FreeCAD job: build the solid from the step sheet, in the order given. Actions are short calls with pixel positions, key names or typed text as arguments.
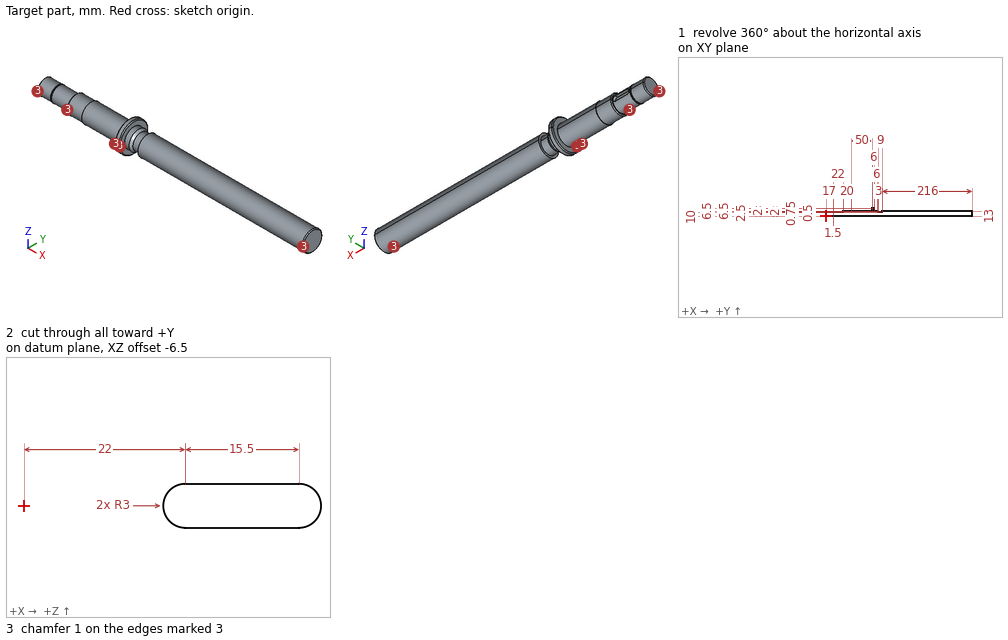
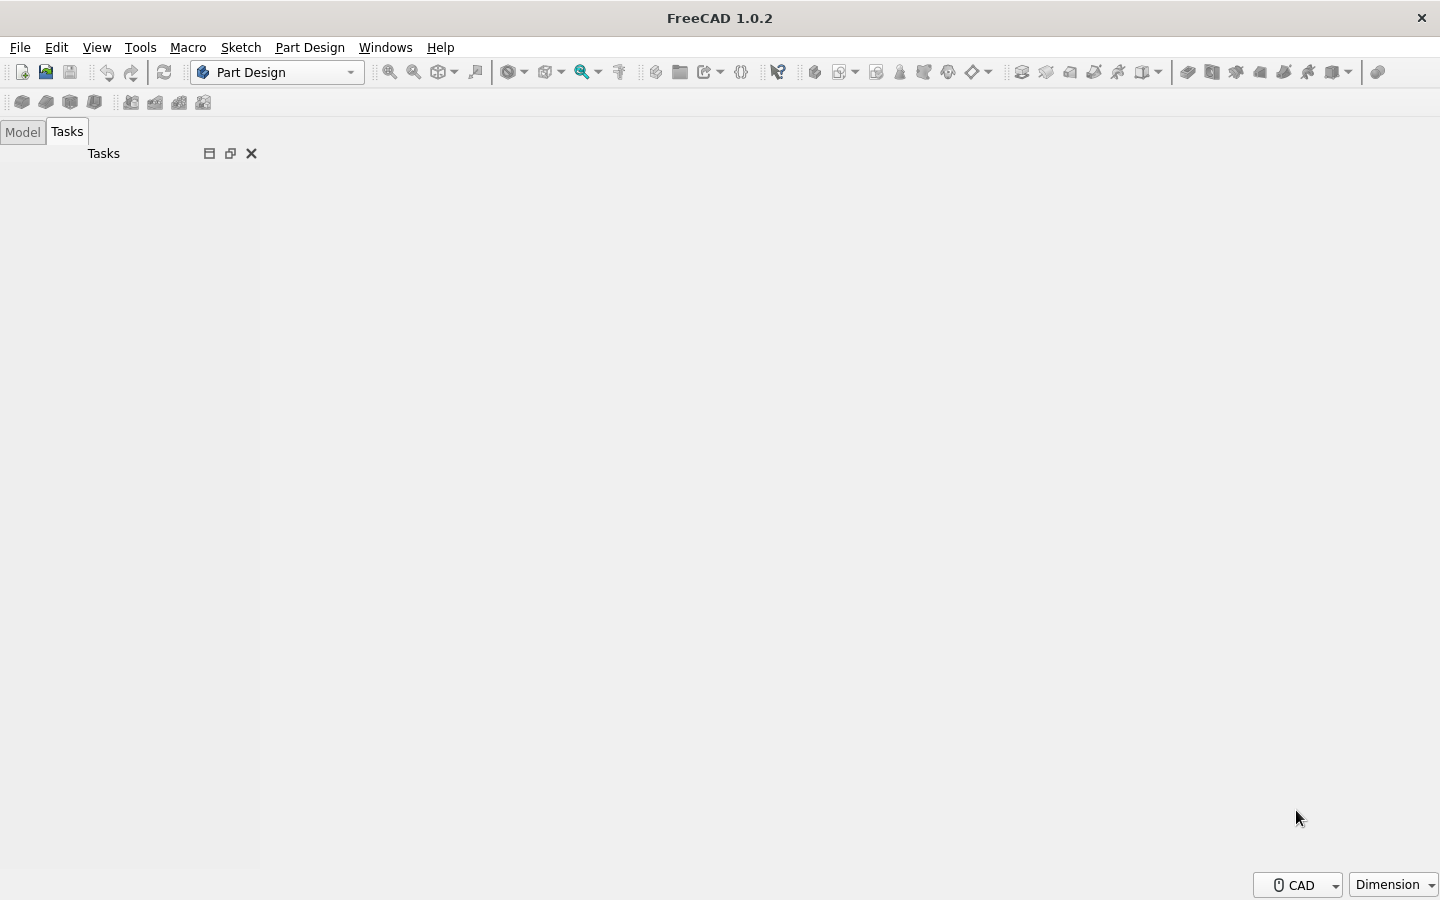
click(22, 72)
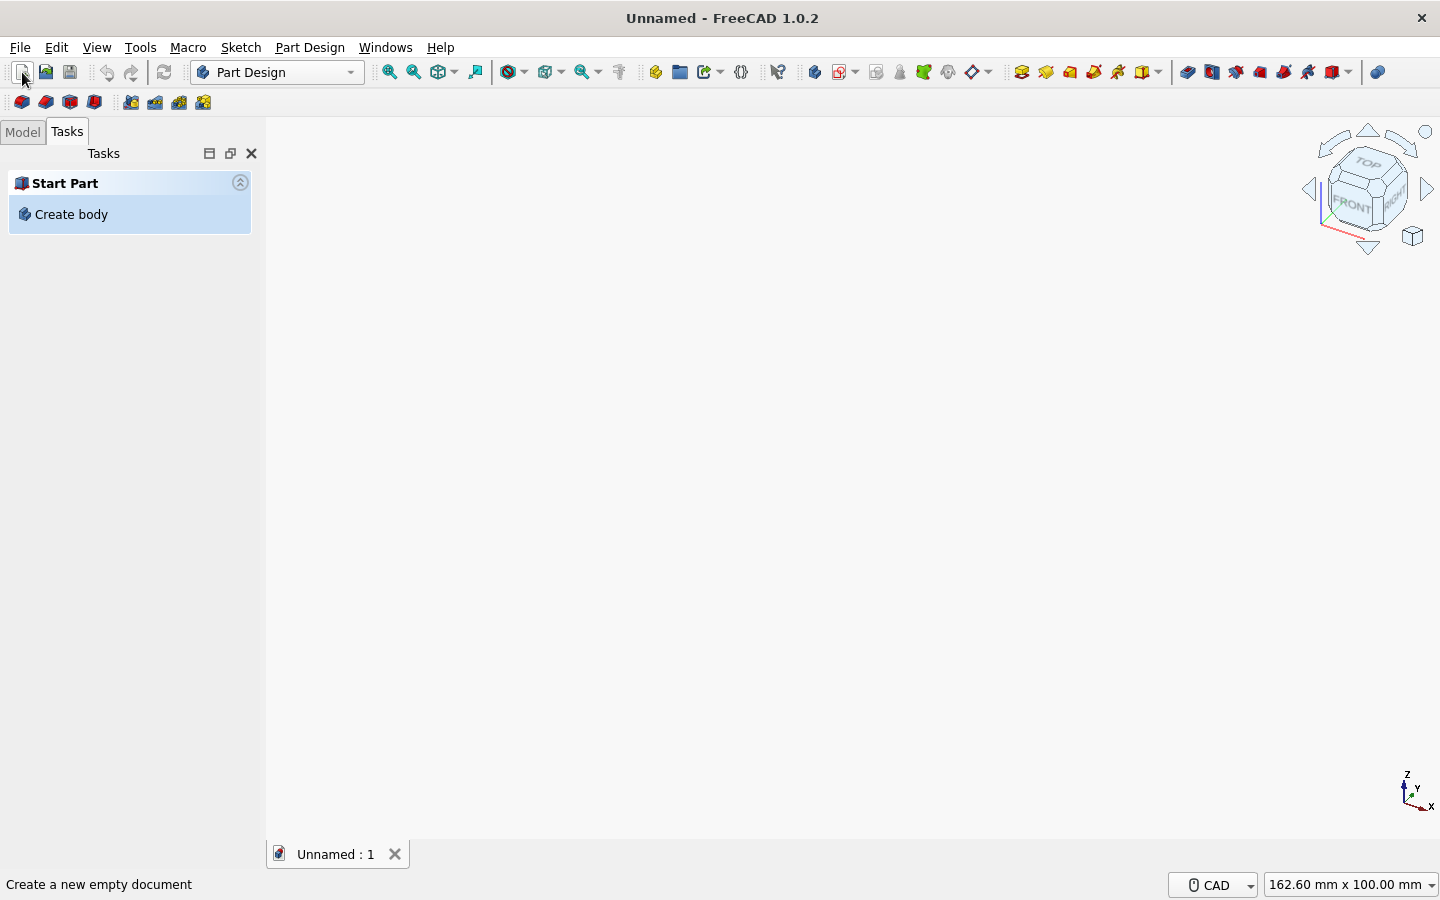
click(840, 72)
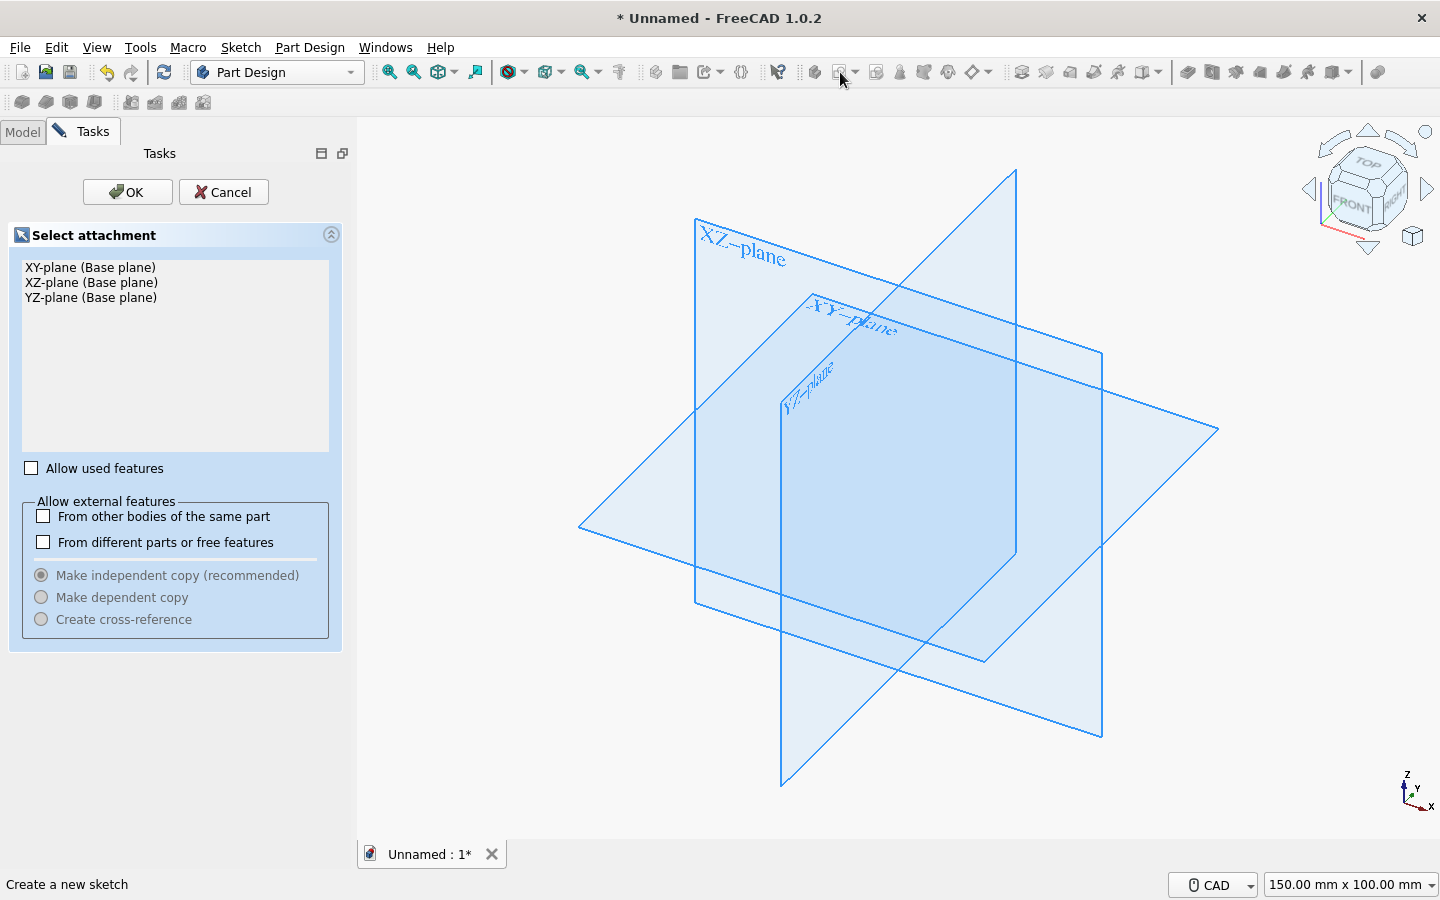
click(82, 268)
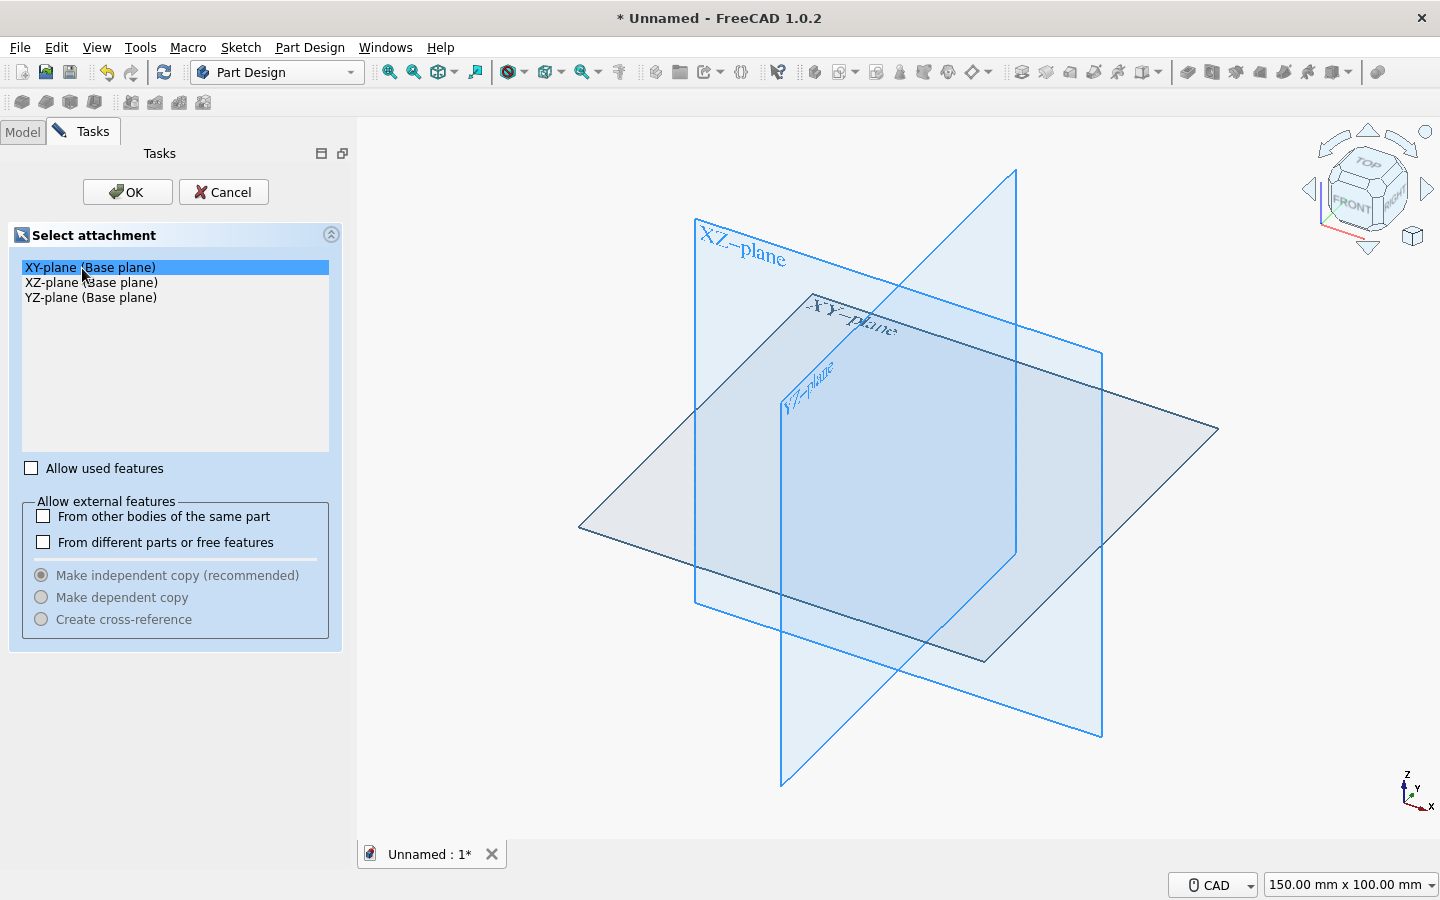
click(128, 192)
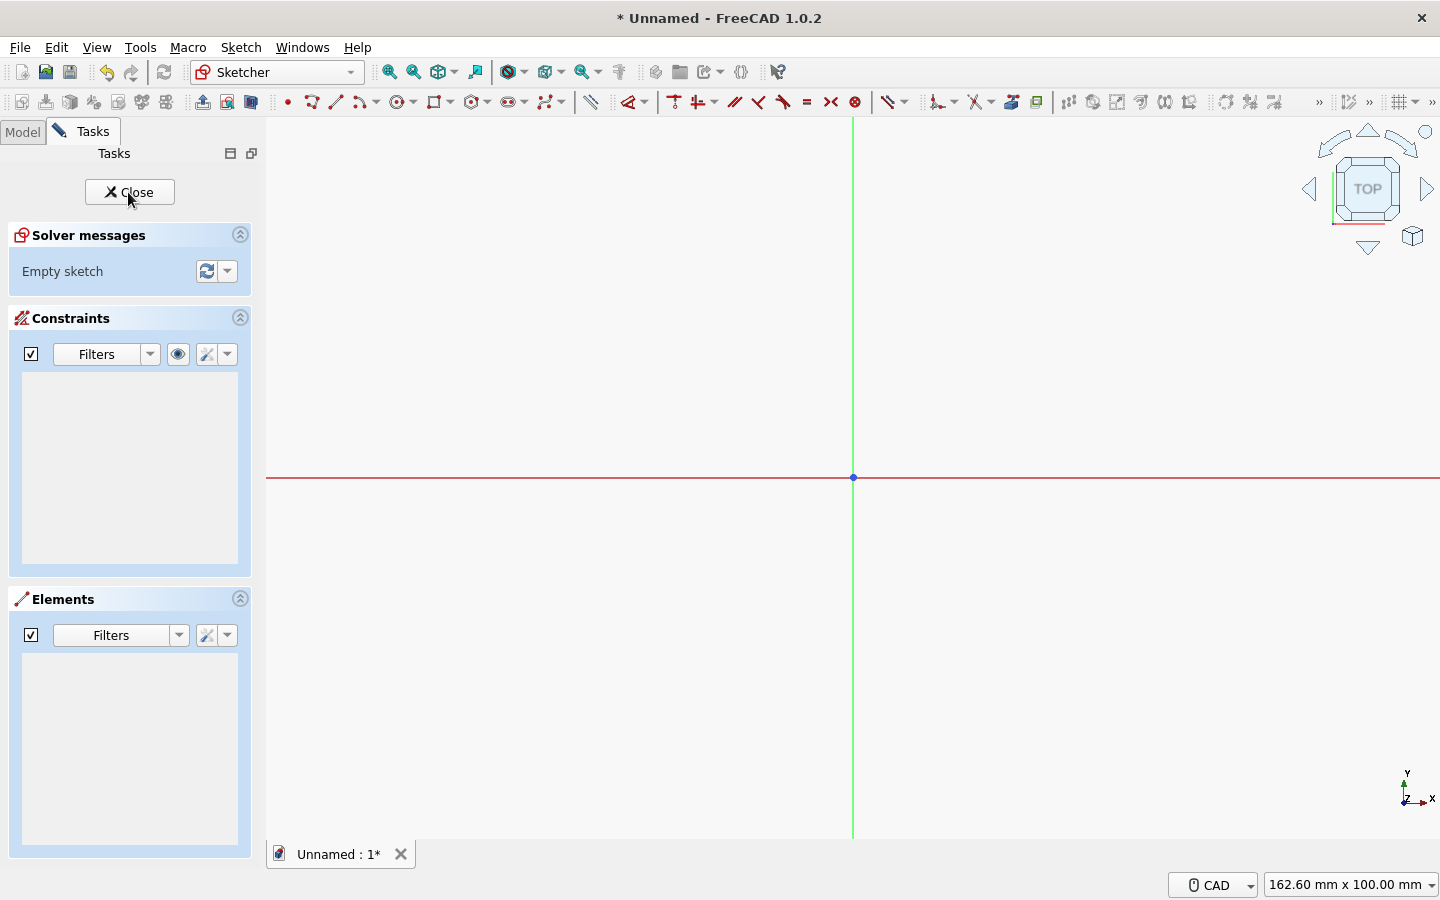
scroll(294, 508, down, 6)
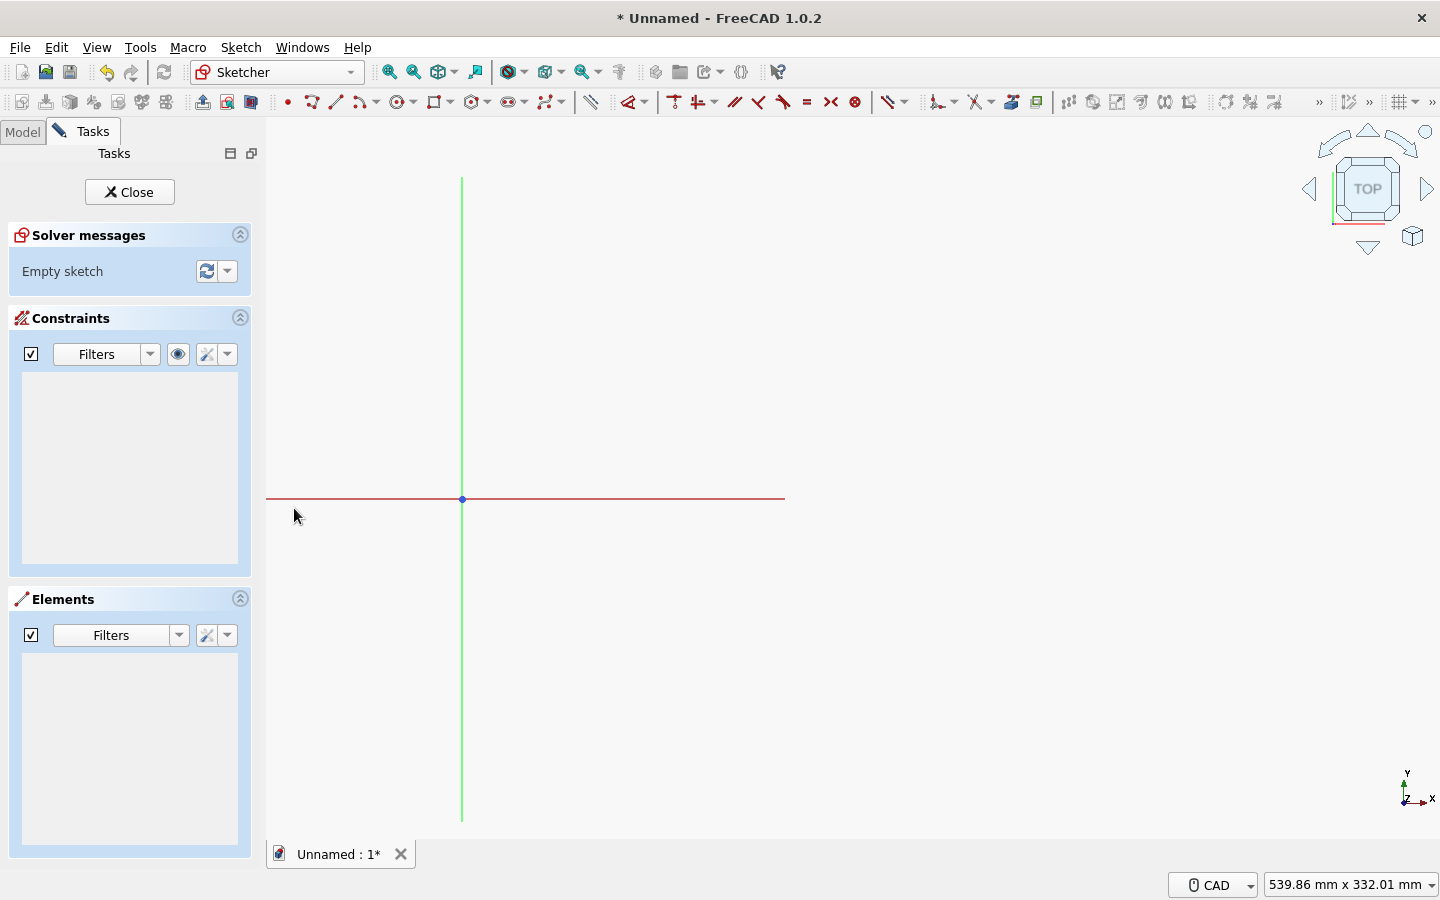
key(g)
key(m)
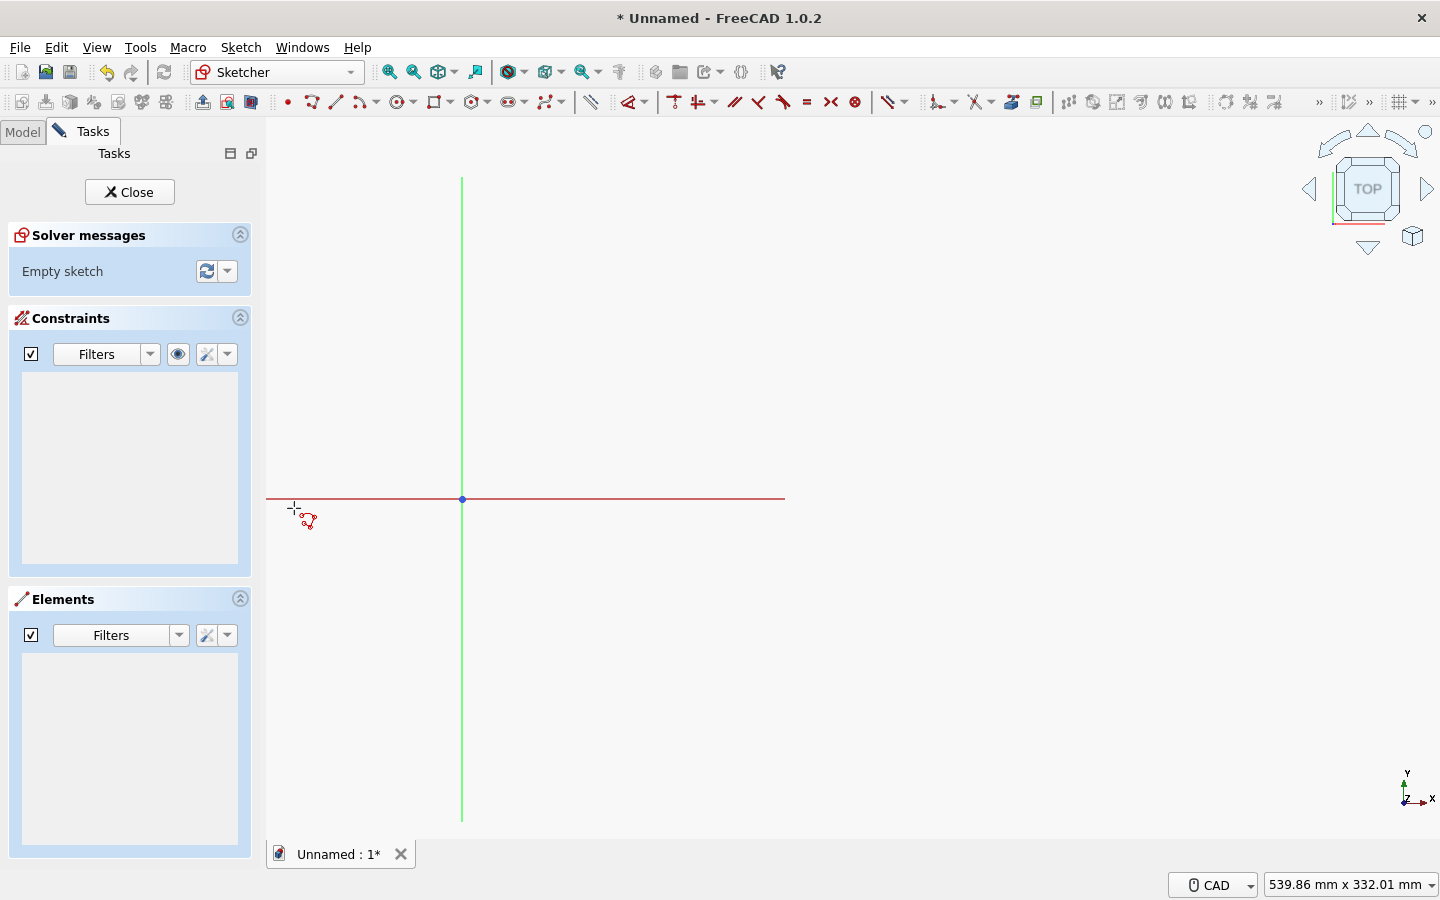
click(462, 499)
click(1225, 490)
click(1225, 471)
click(755, 471)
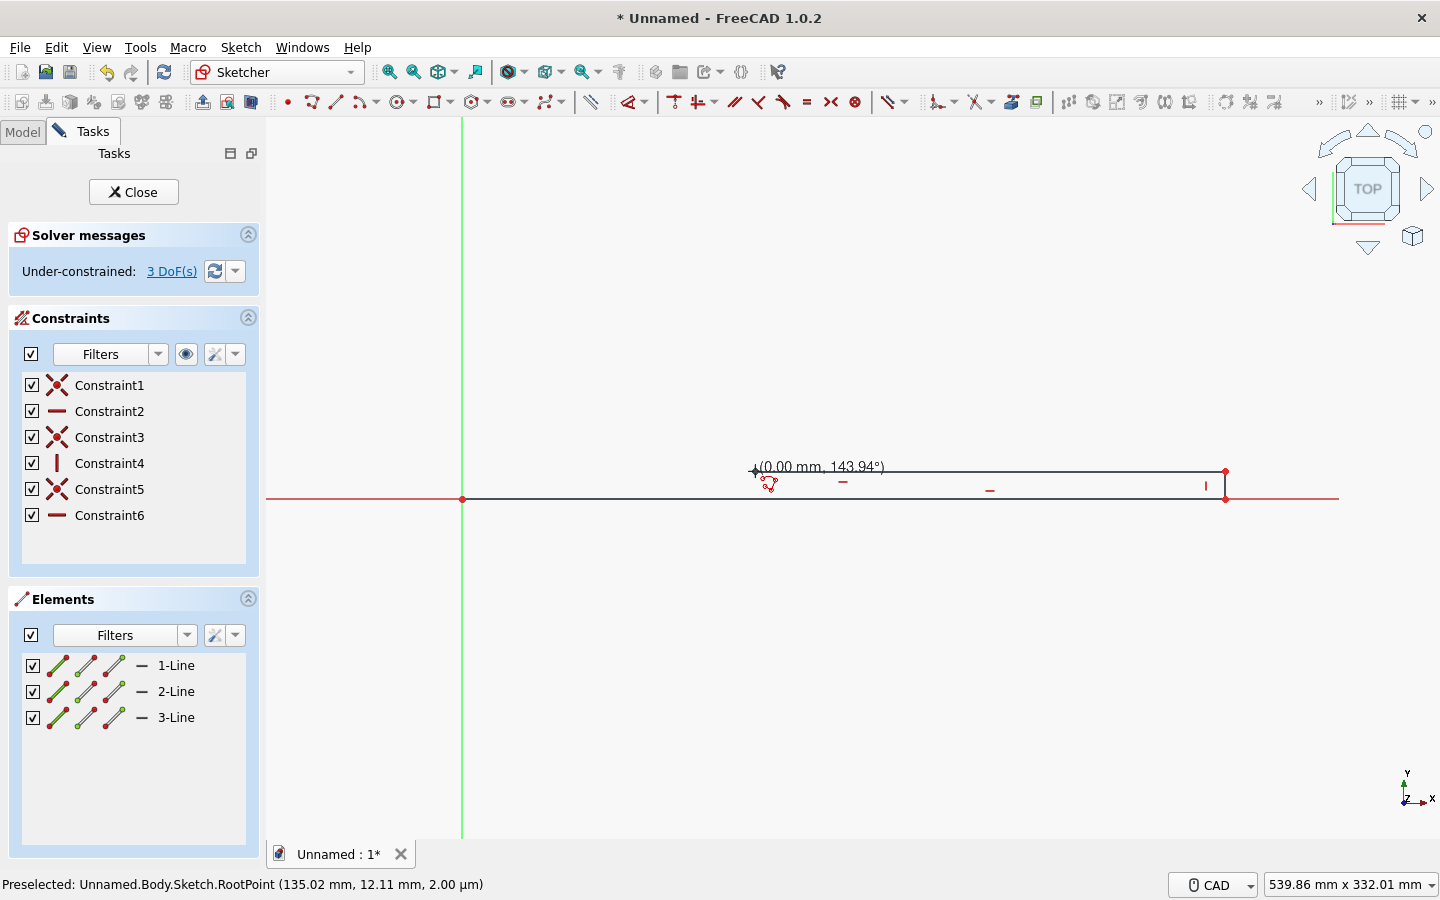
scroll(755, 477, up, 6)